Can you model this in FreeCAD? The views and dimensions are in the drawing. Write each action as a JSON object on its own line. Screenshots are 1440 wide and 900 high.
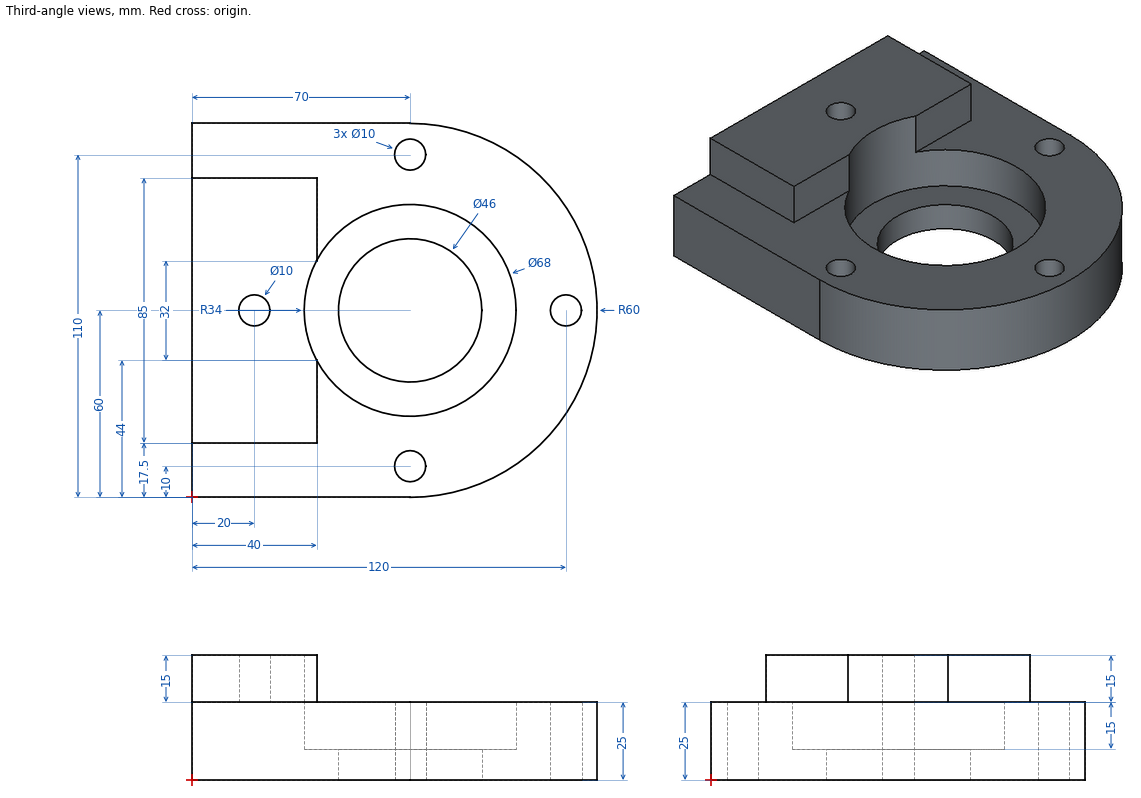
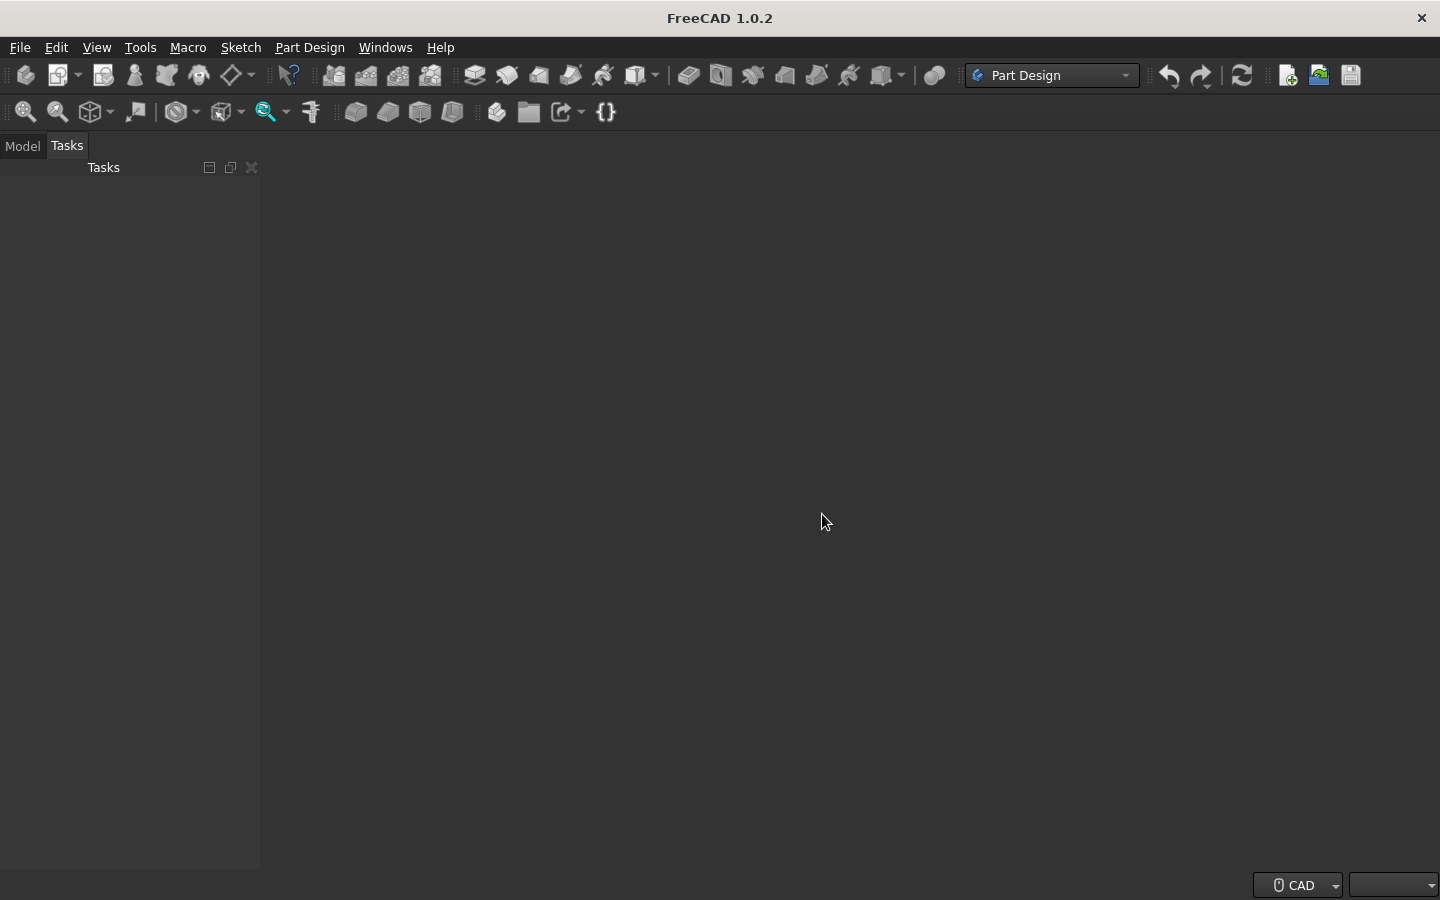
{"action": "left_click", "coordinate": [1288, 76]}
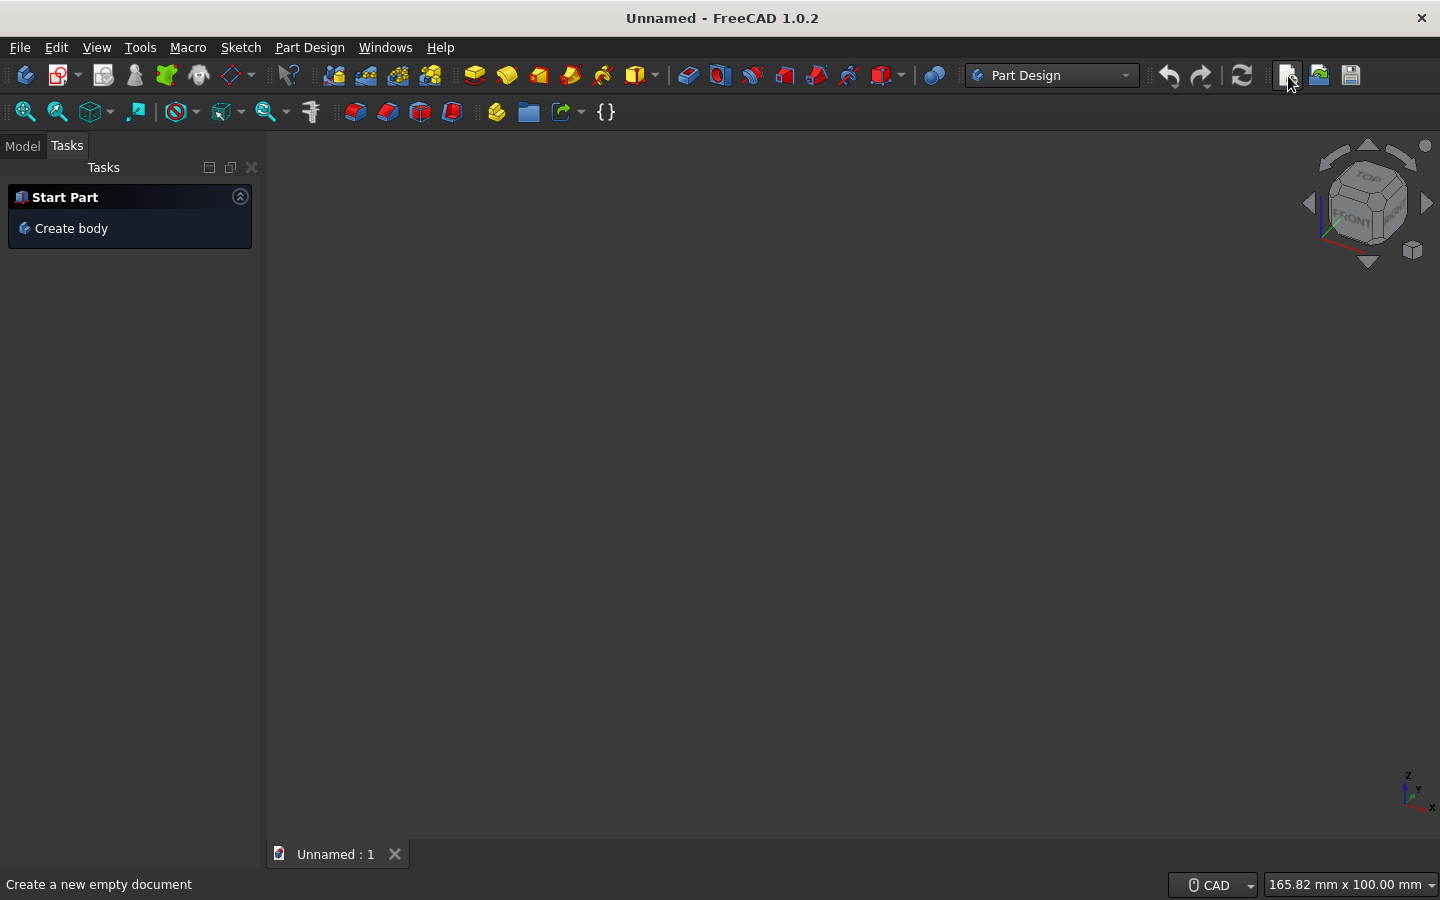
{"action": "left_click", "coordinate": [58, 76]}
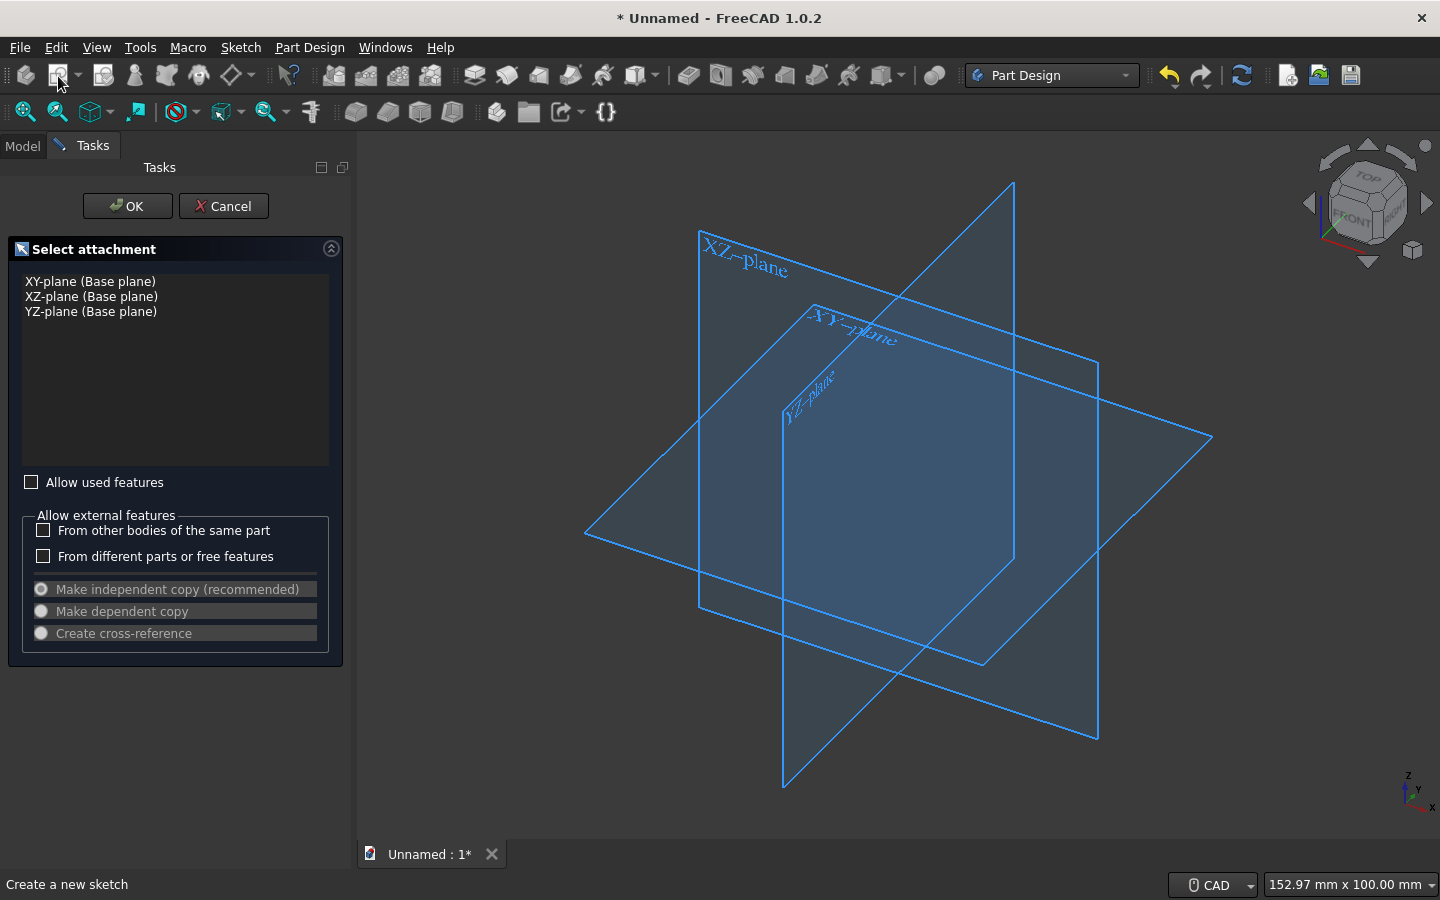
{"action": "left_click", "coordinate": [82, 282]}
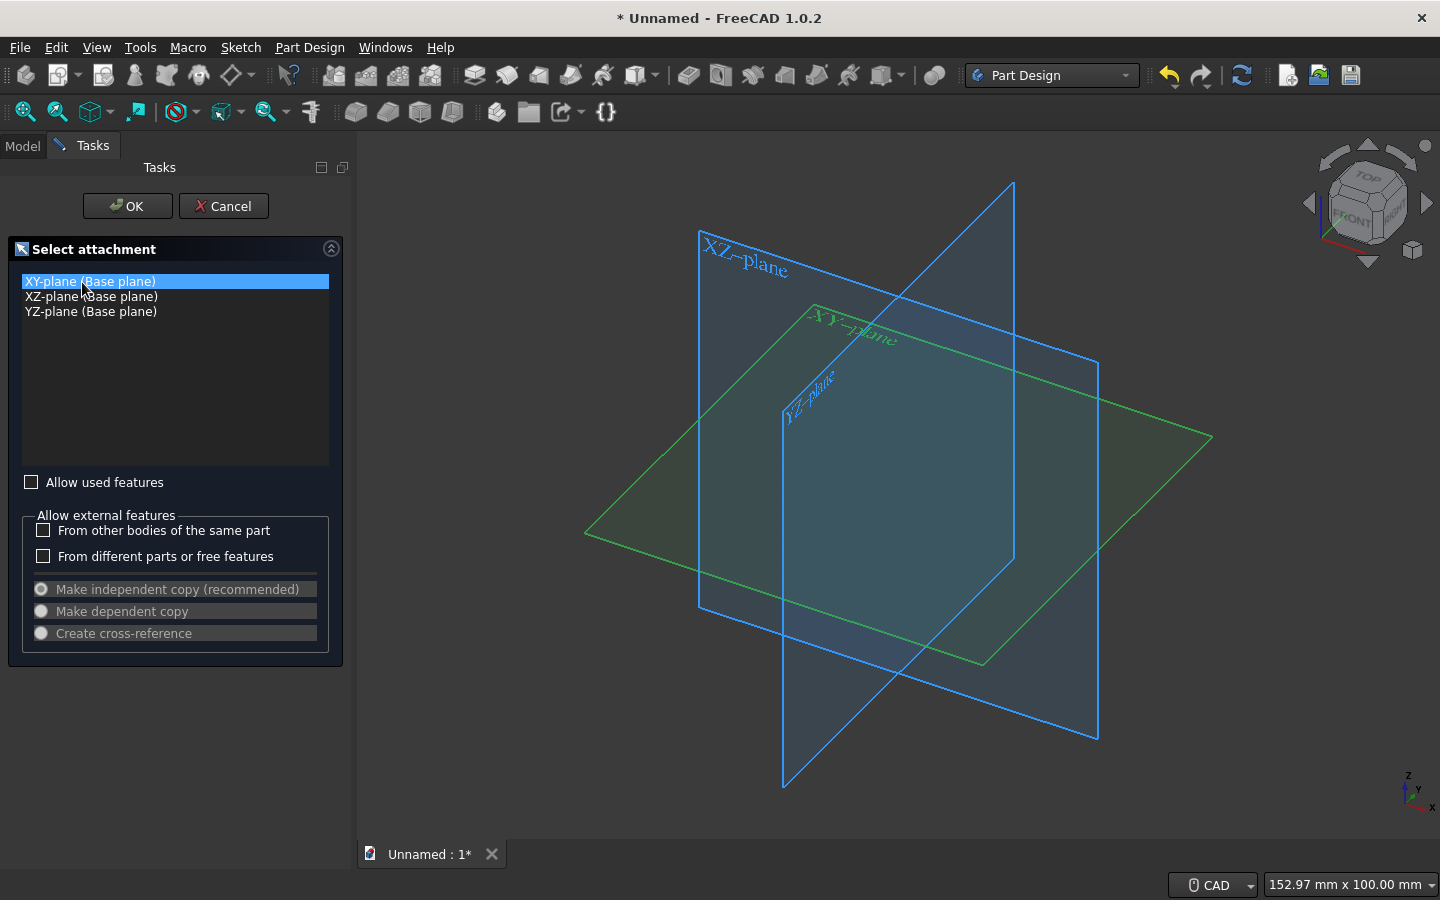
{"action": "left_click", "coordinate": [128, 206]}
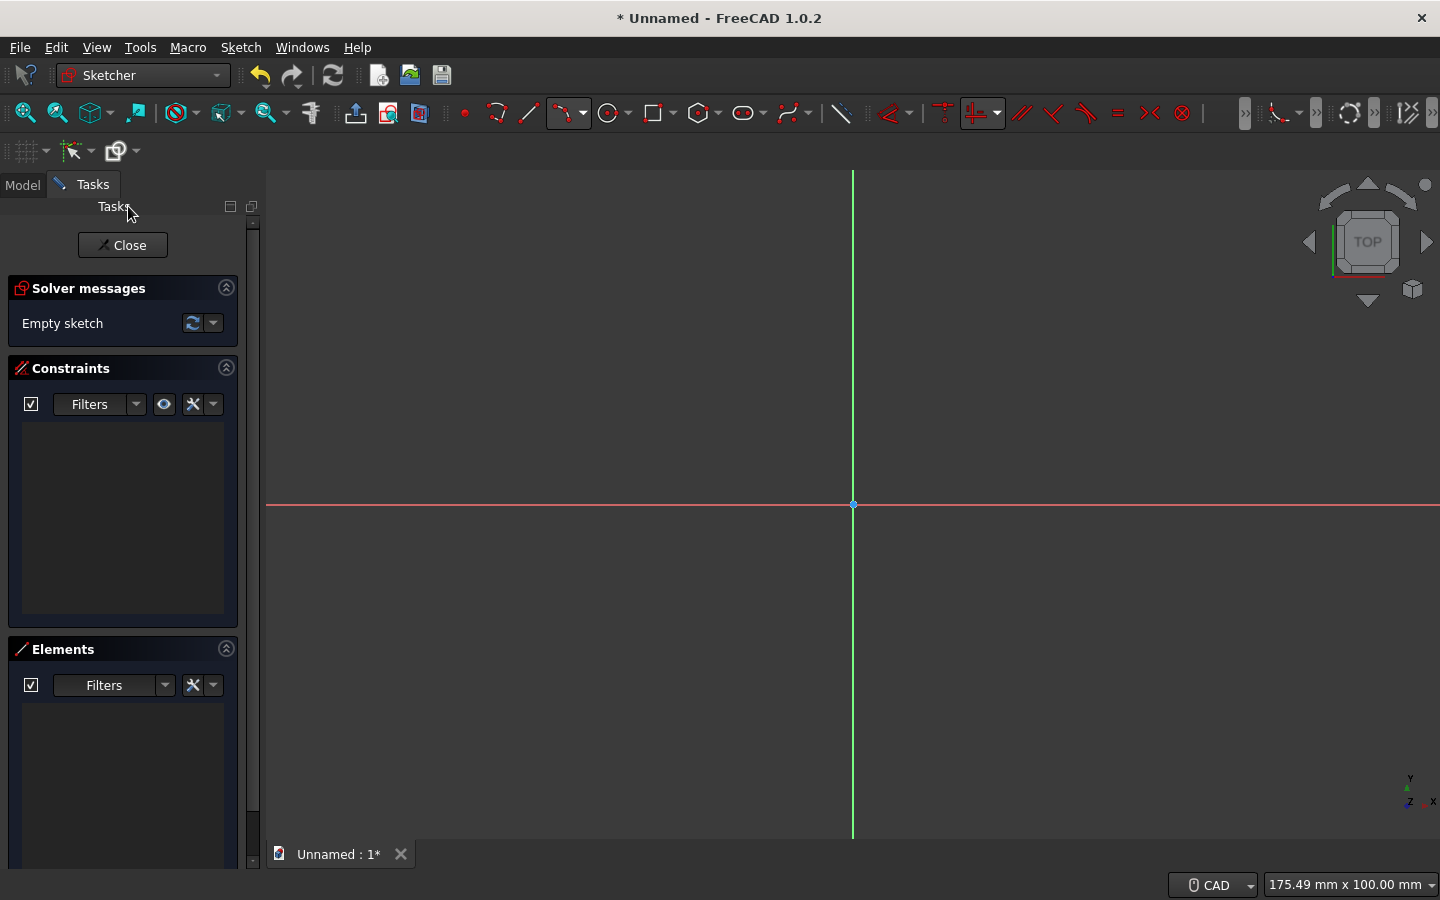
{"action": "scroll", "coordinate": [374, 811], "scroll_direction": "down", "scroll_amount": 4}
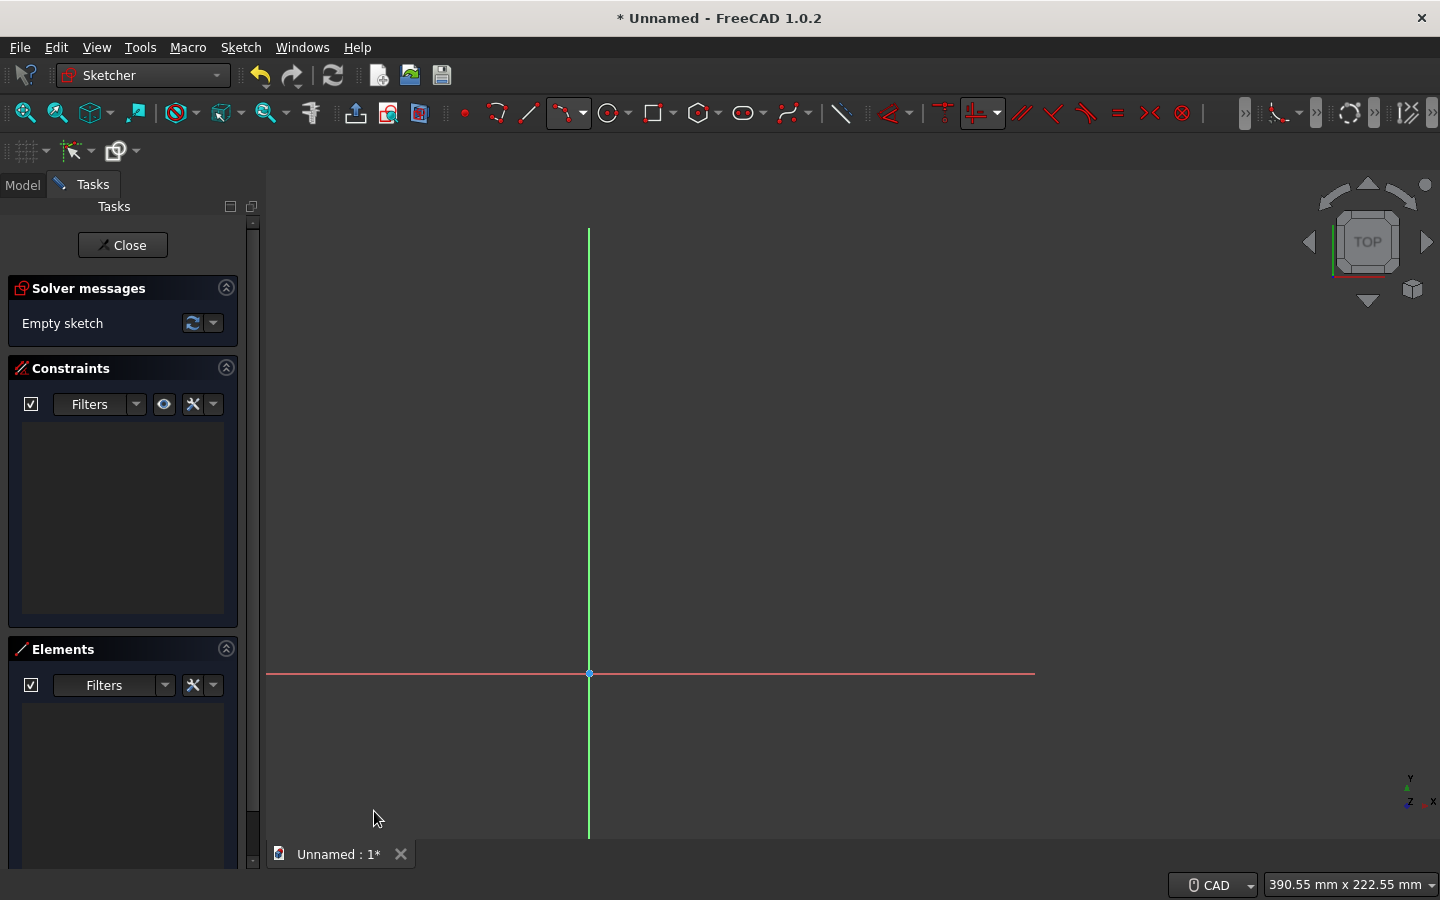
{"action": "key", "text": "g m"}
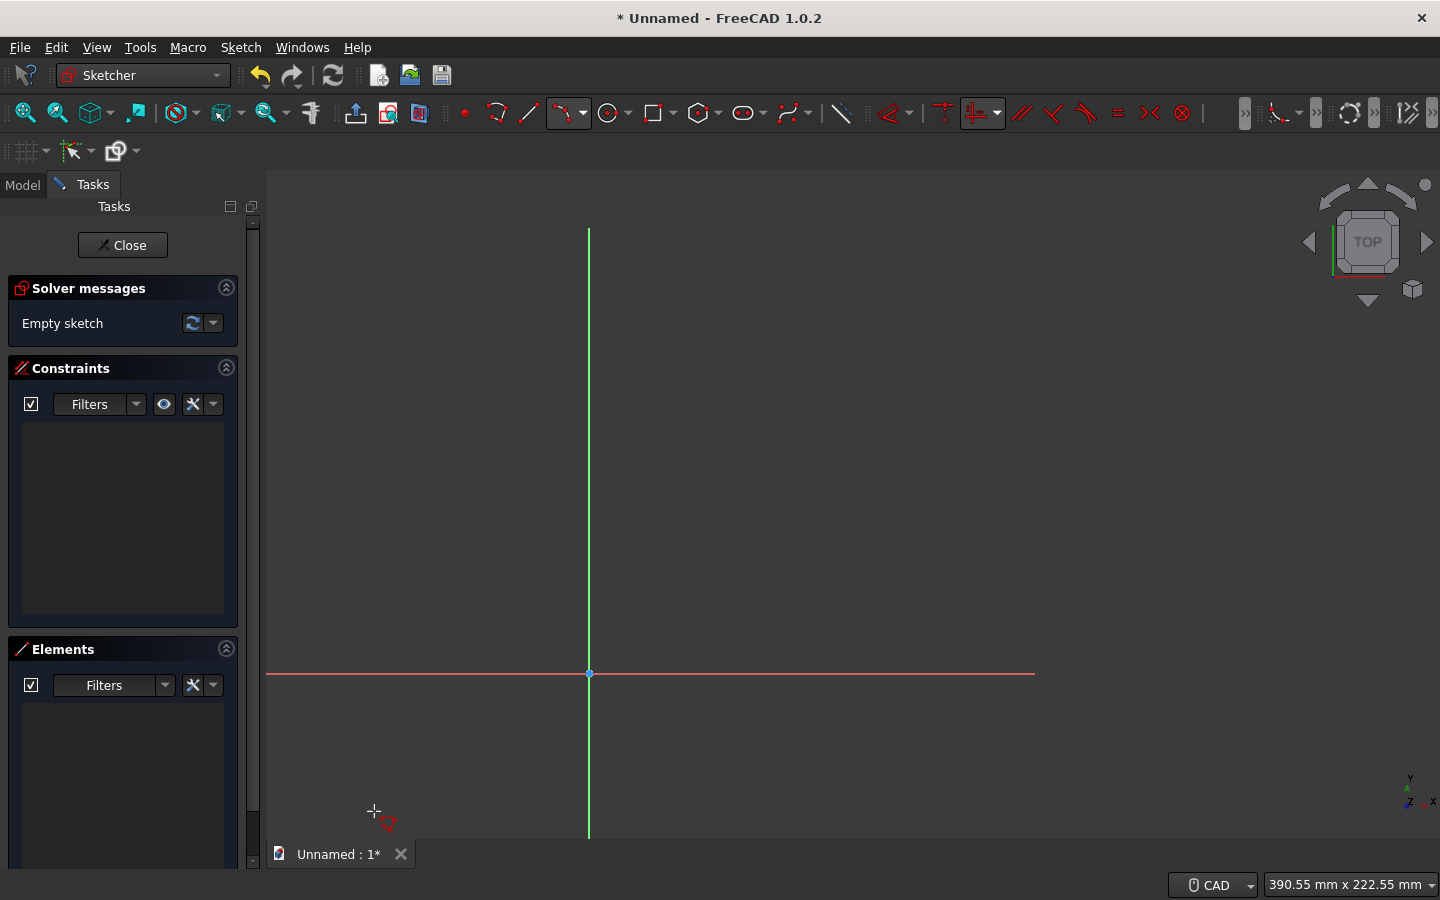
{"action": "left_click", "coordinate": [800, 313]}
{"action": "left_click", "coordinate": [589, 313]}
{"action": "left_click", "coordinate": [589, 674]}
{"action": "left_click", "coordinate": [800, 665]}
{"action": "right_click", "coordinate": [800, 665]}